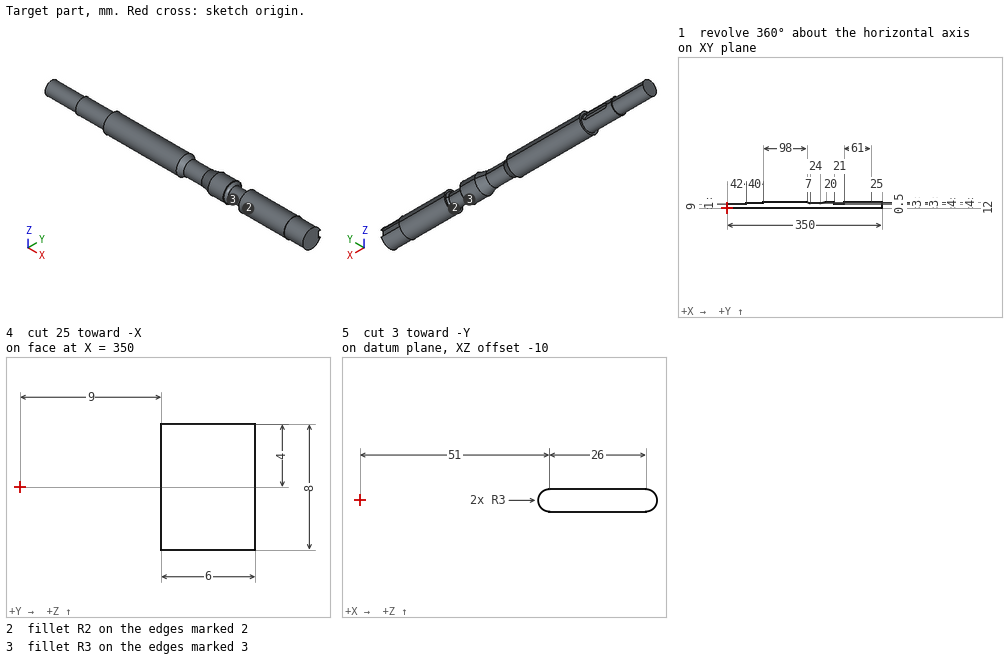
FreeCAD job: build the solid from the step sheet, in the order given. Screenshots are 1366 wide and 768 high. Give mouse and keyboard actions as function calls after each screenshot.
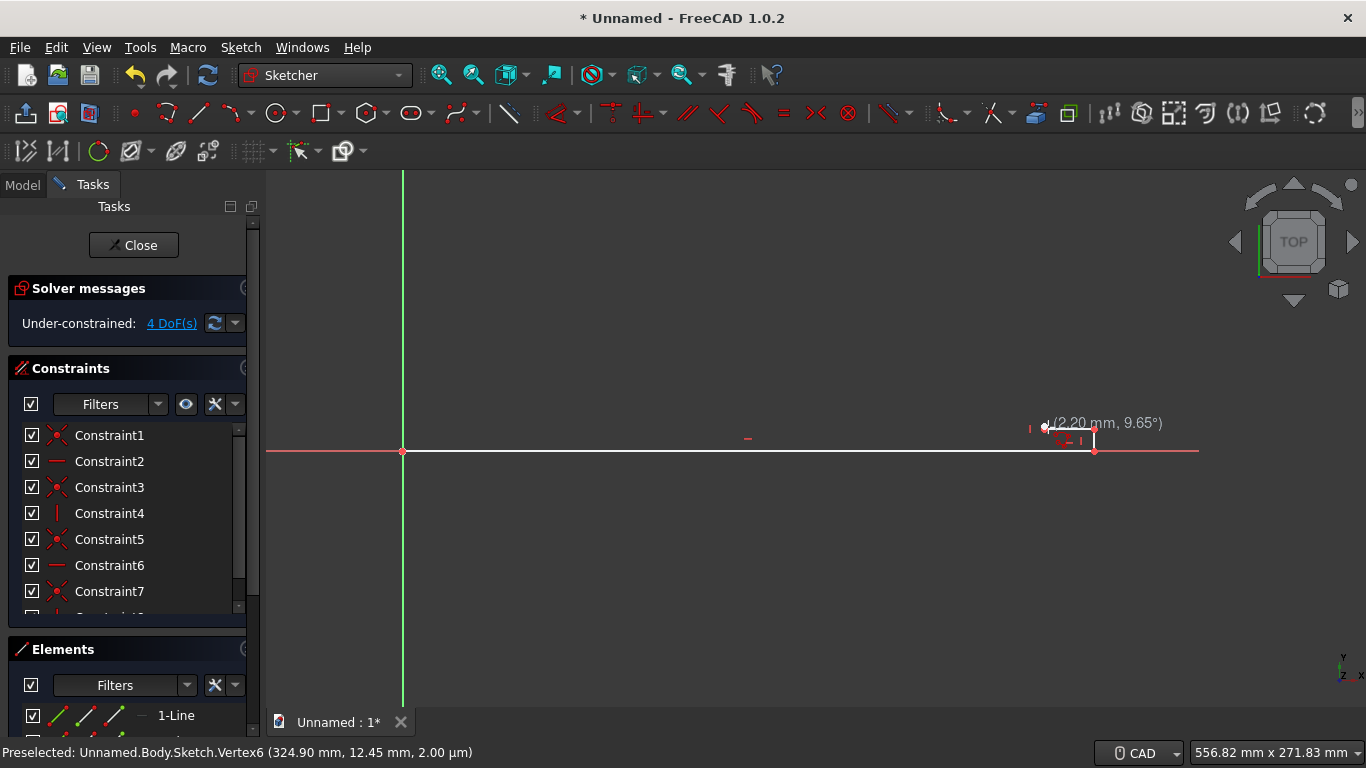
click(924, 427)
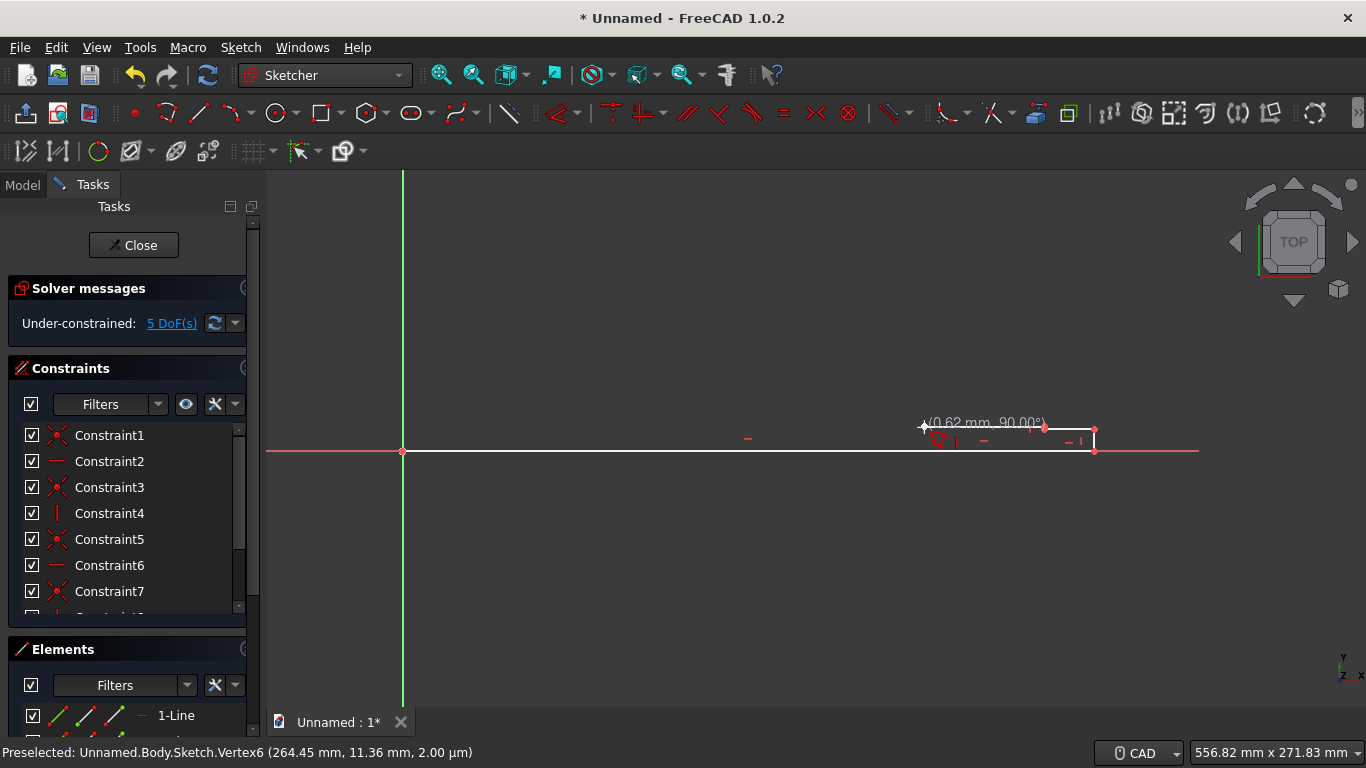
scroll(924, 435, up, 4)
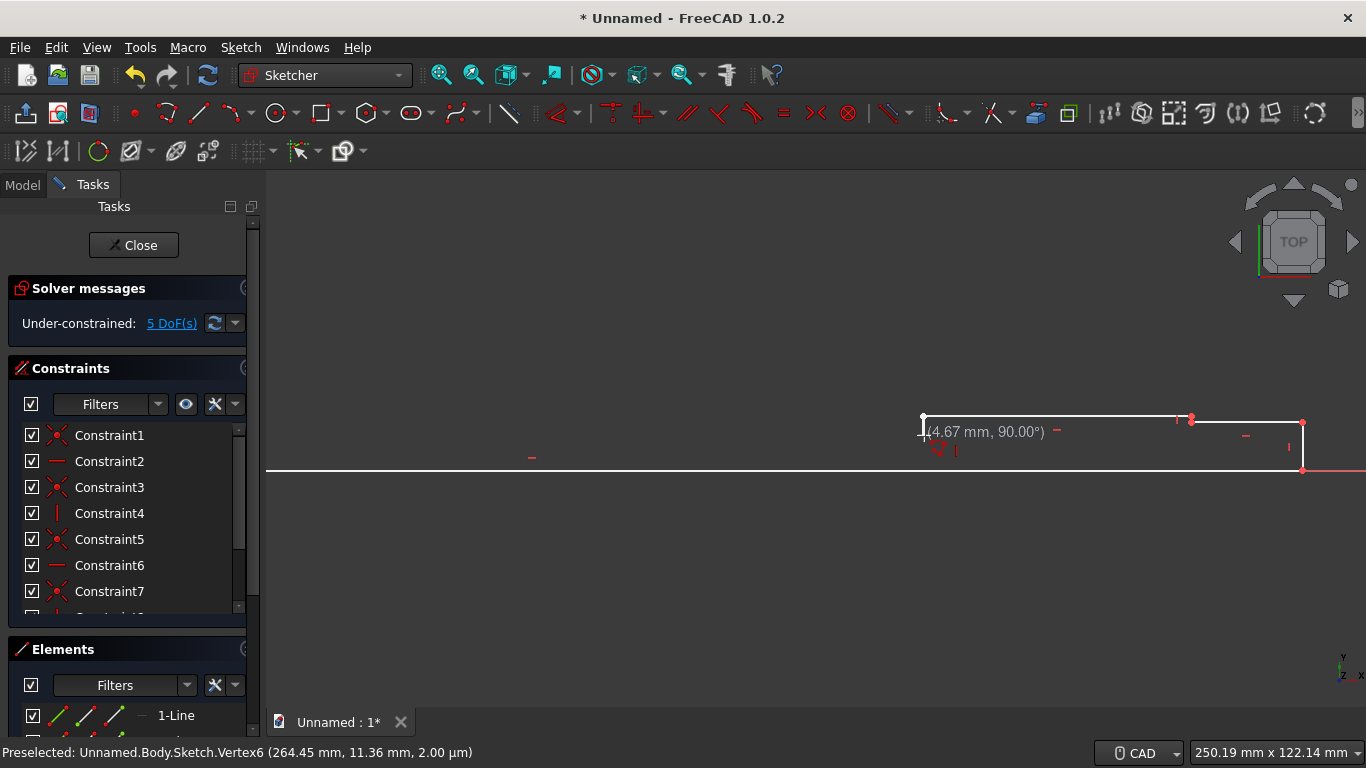
click(923, 434)
click(831, 434)
click(831, 416)
click(743, 416)
click(690, 429)
click(585, 429)
click(554, 416)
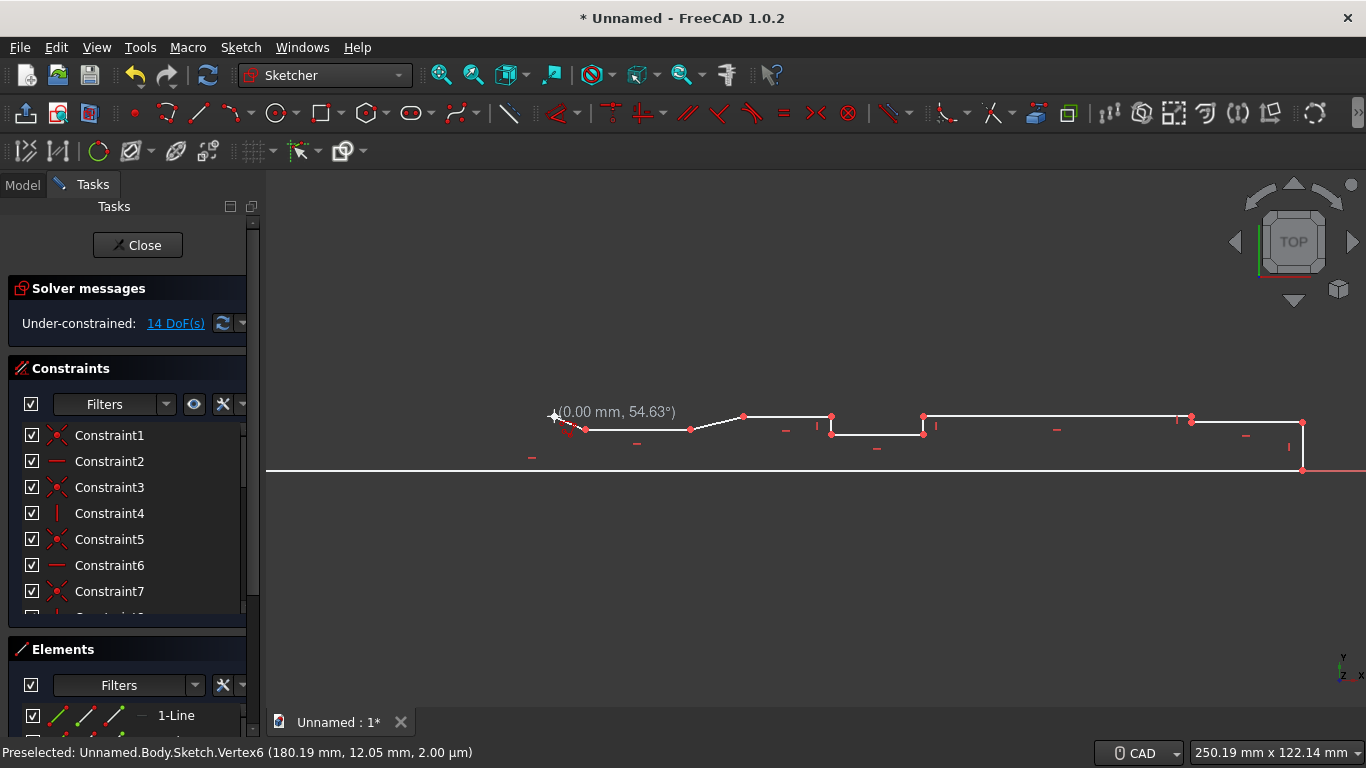
scroll(923, 434, down, 4)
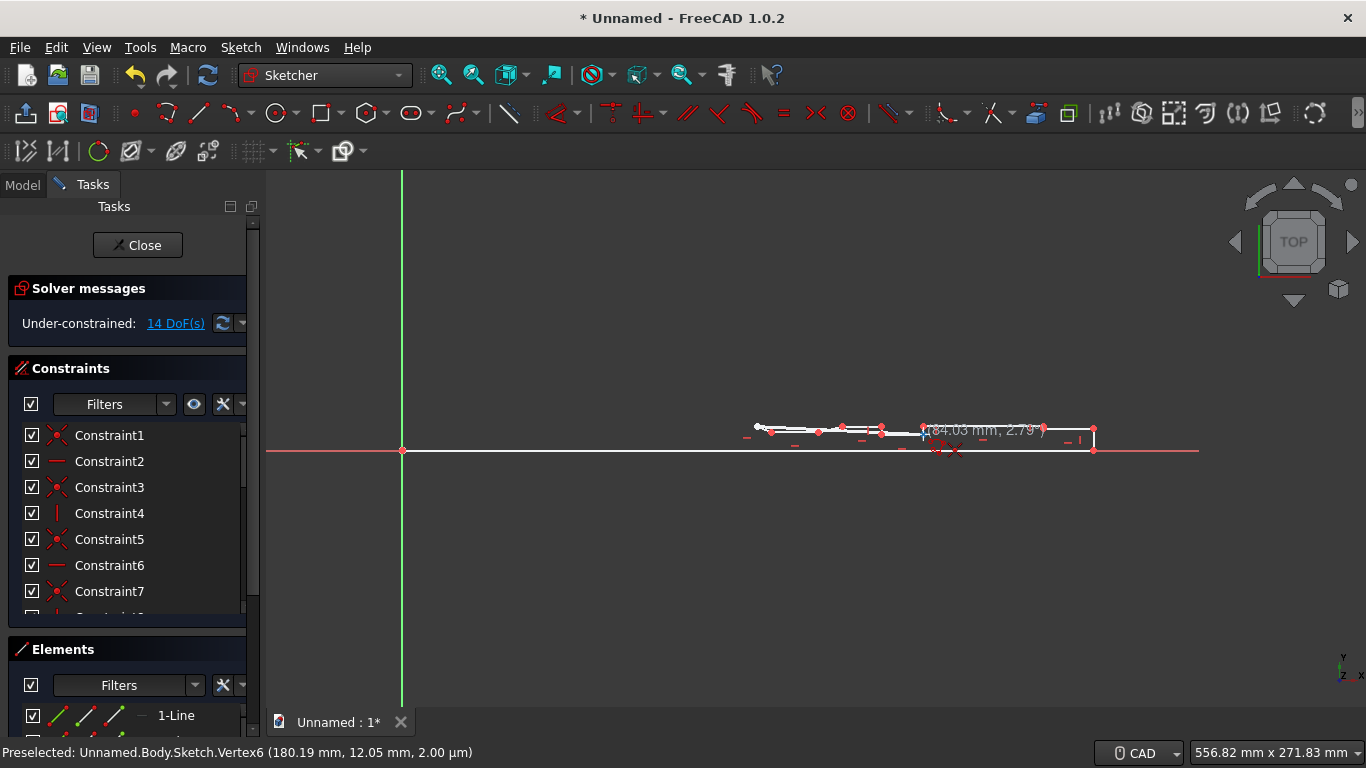
click(564, 426)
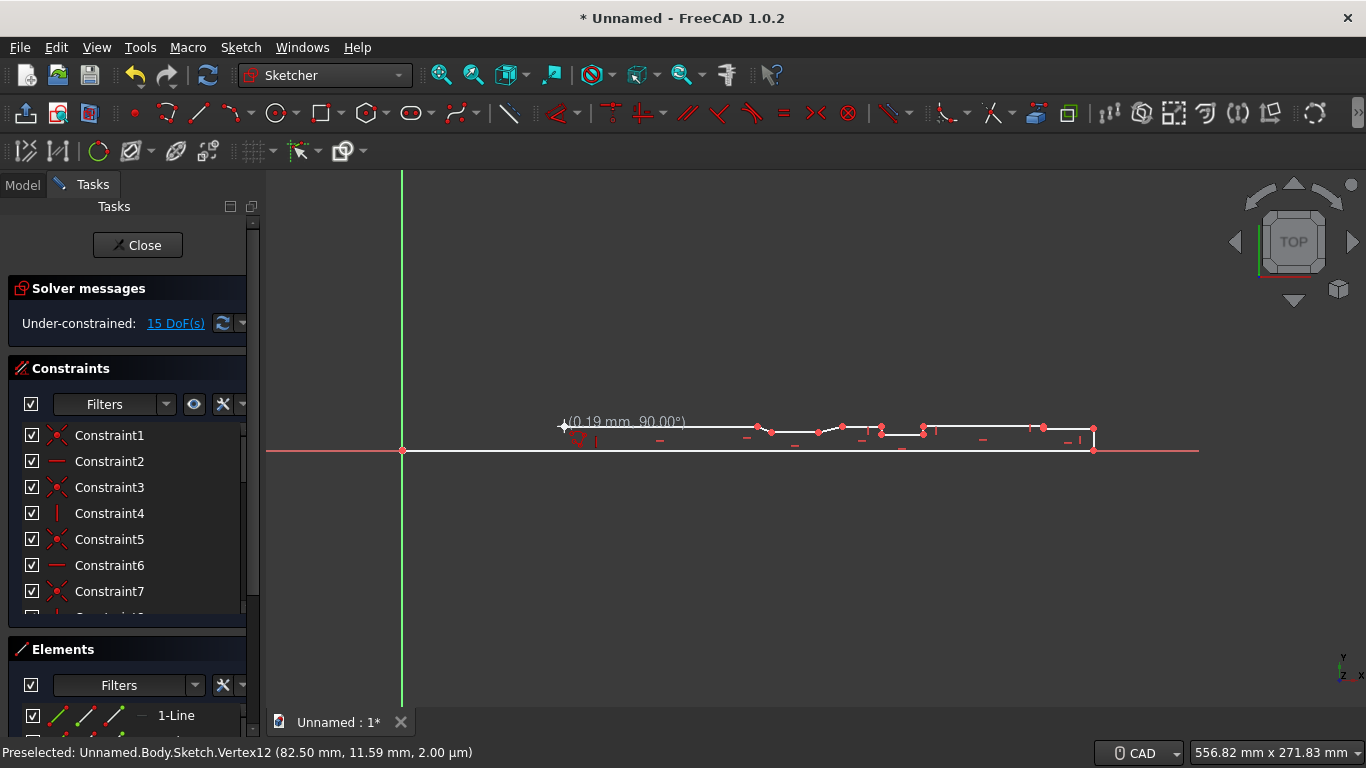
scroll(564, 431, up, 6)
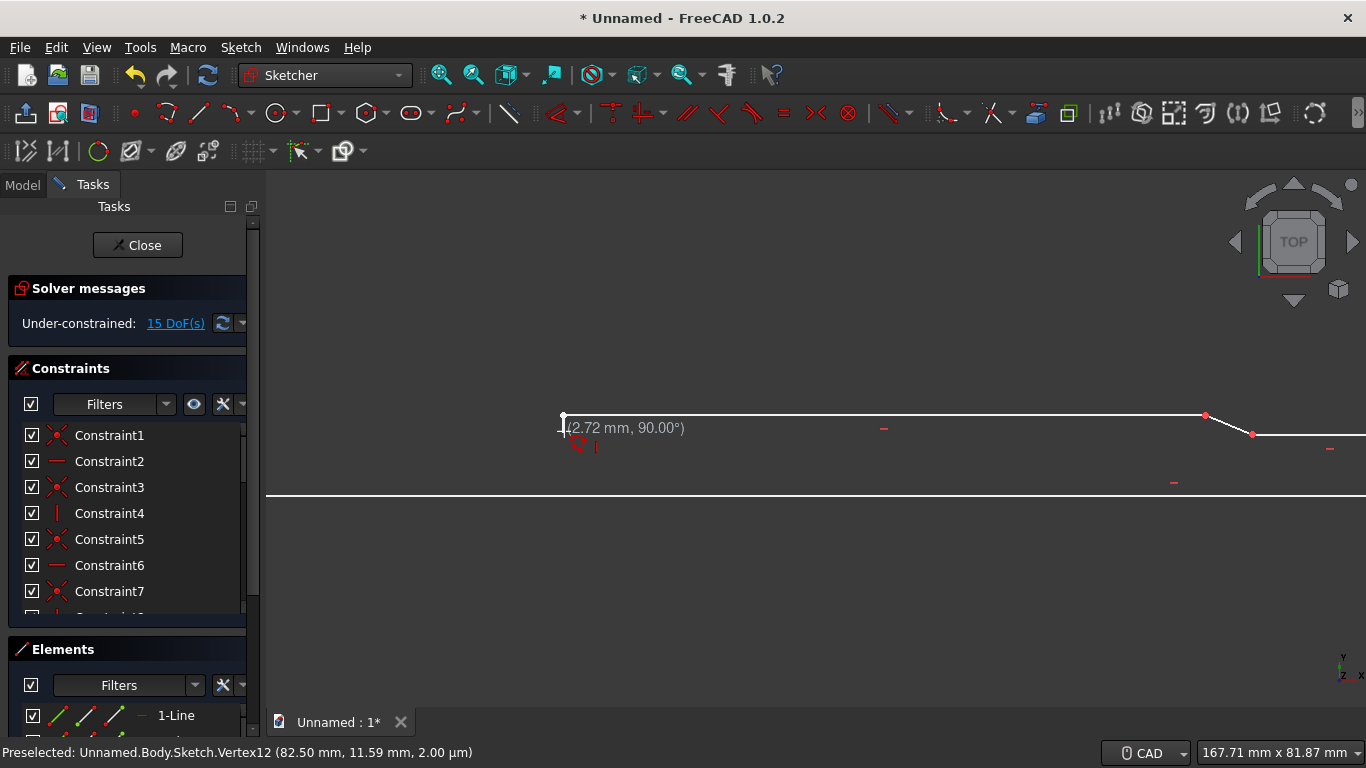
click(563, 430)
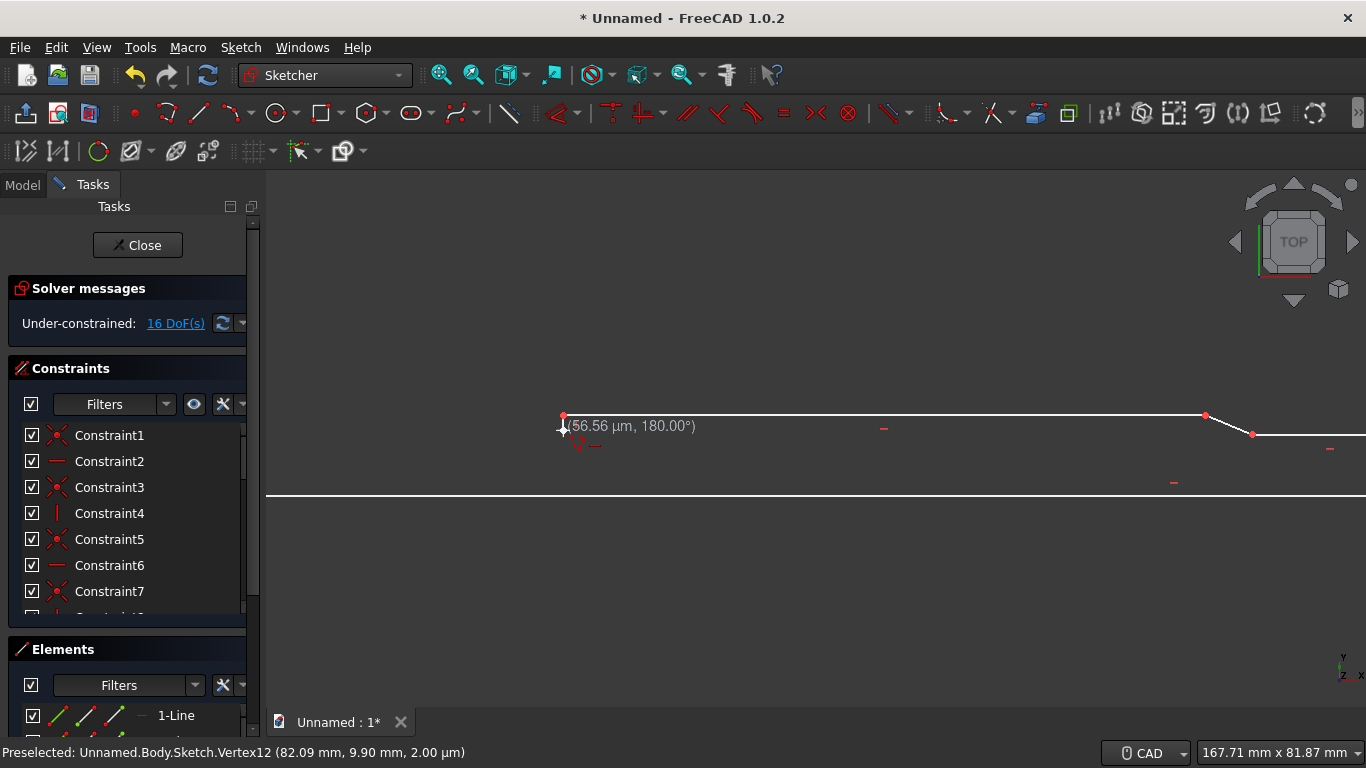
scroll(564, 431, down, 6)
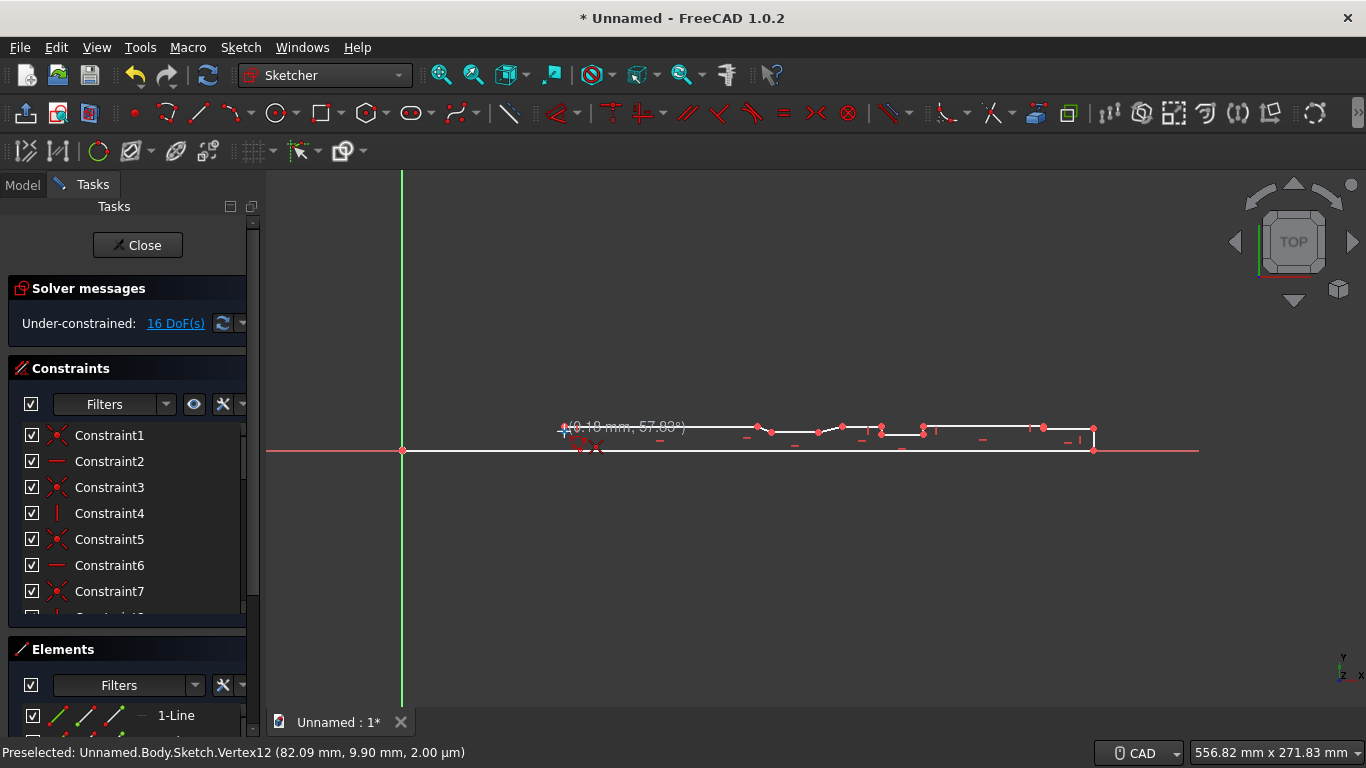
click(485, 431)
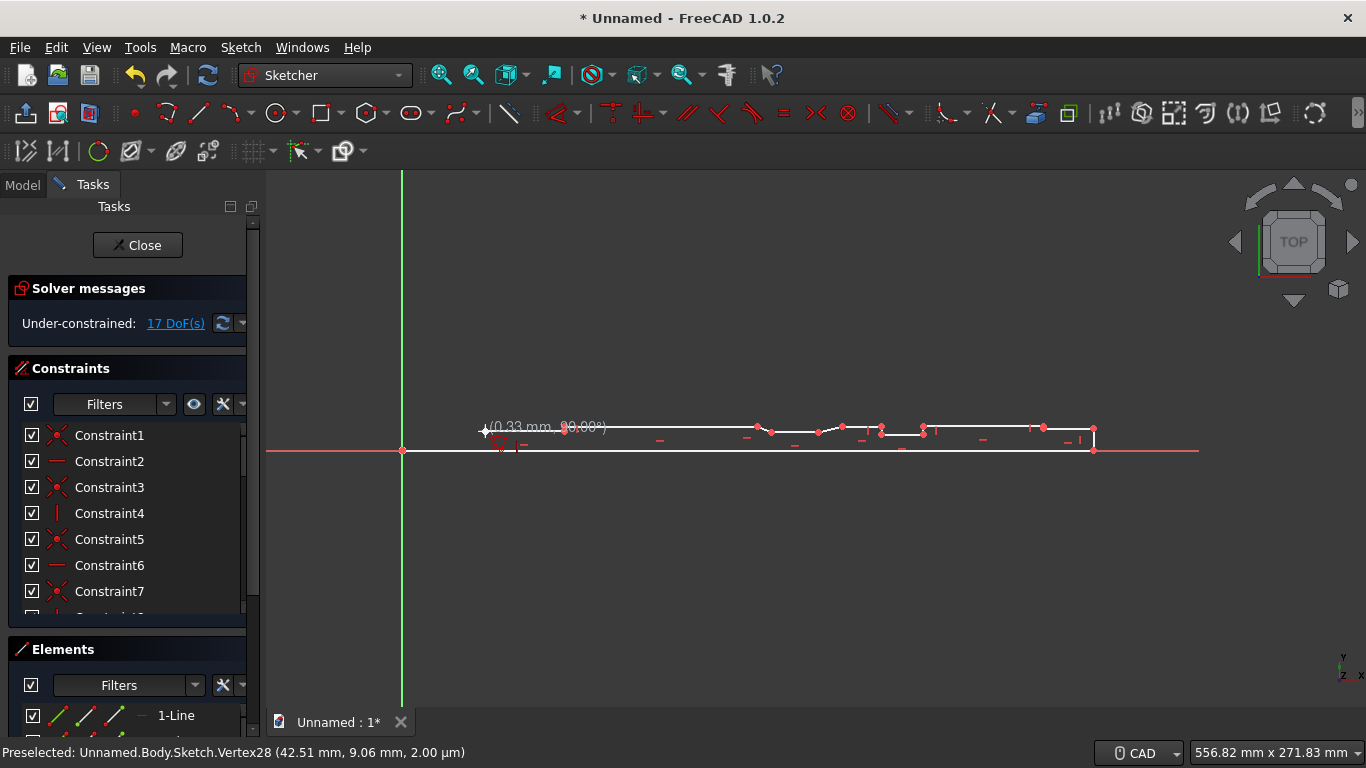
scroll(485, 433, up, 11)